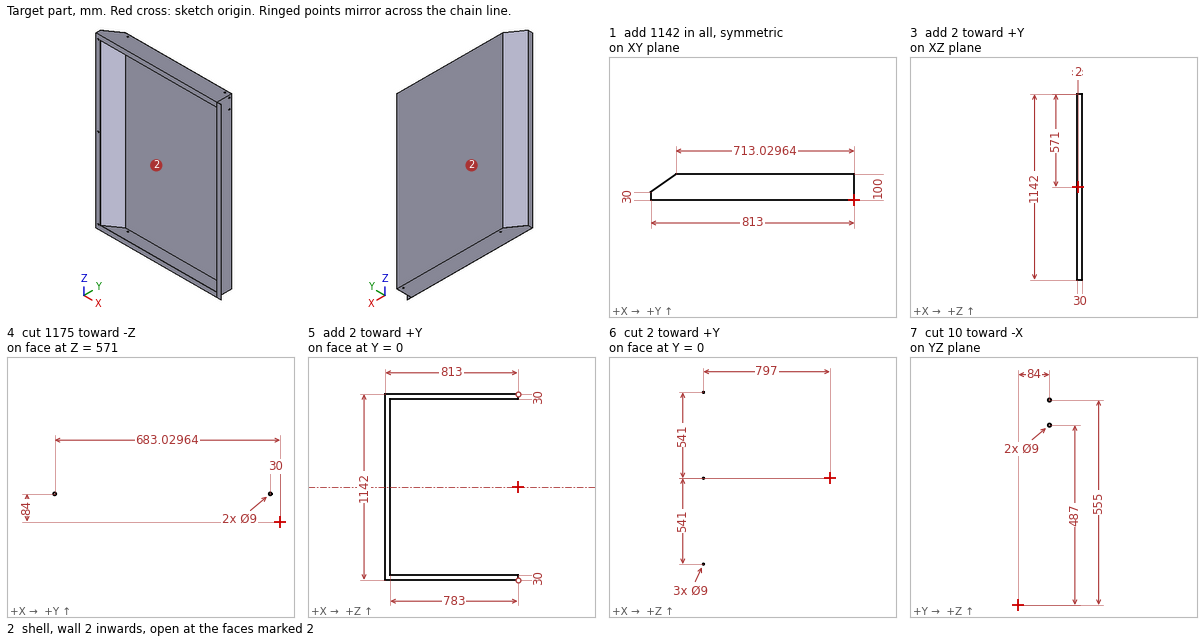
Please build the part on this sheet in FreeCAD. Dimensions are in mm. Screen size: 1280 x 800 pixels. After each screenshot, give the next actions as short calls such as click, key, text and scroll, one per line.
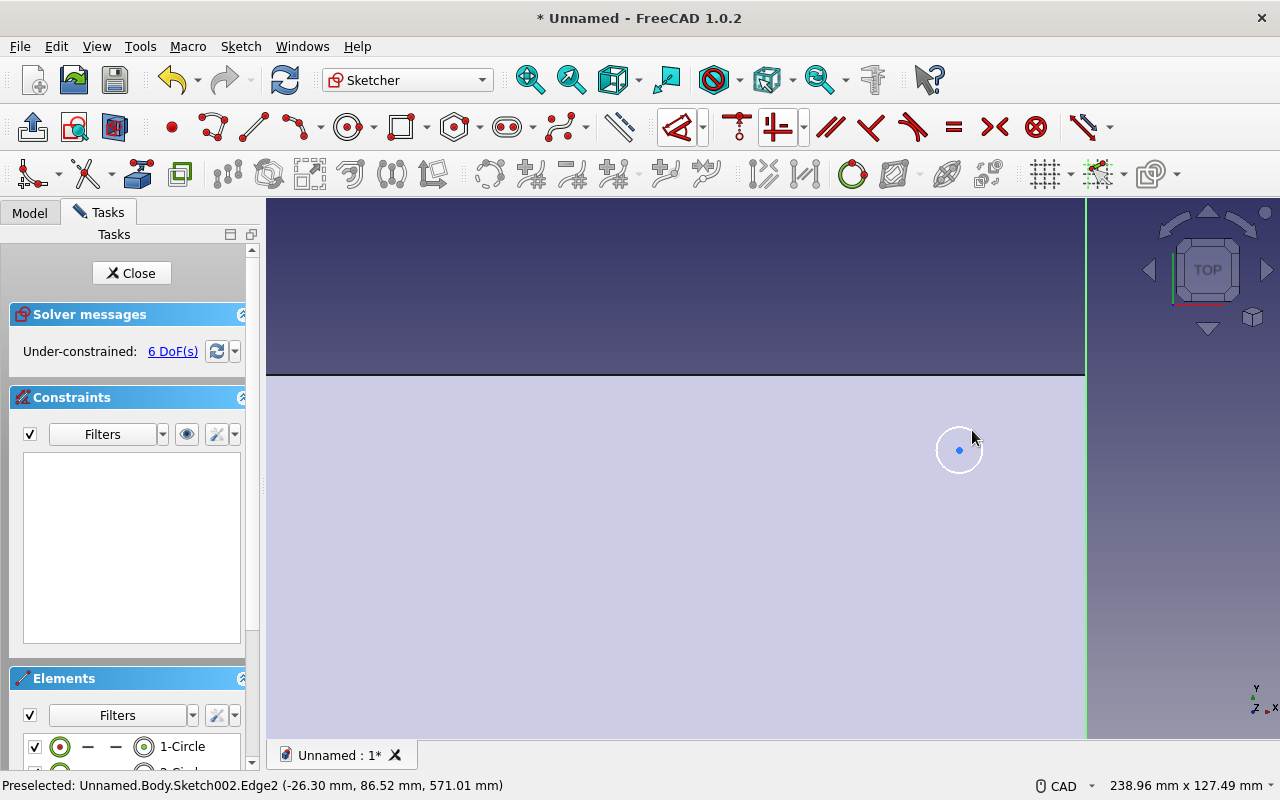
scroll(977, 432, down, 8)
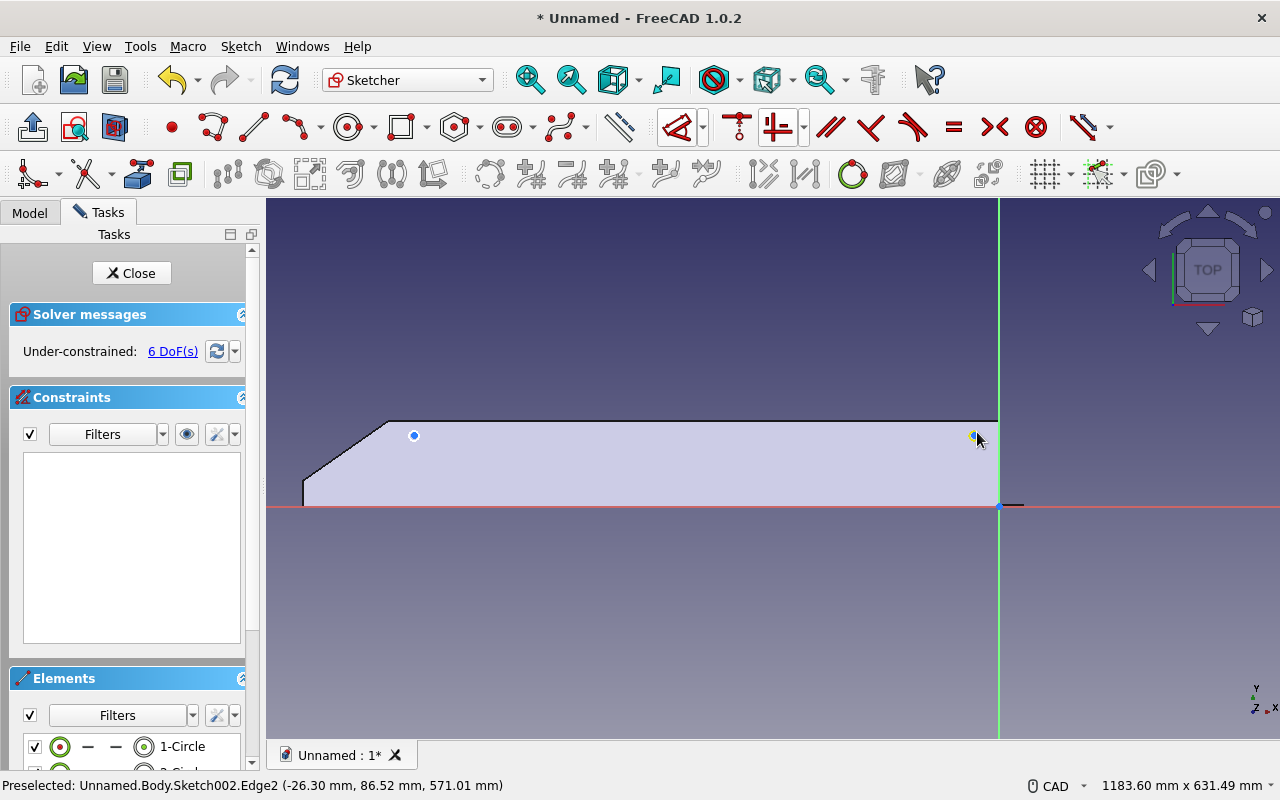
scroll(417, 432, up, 6)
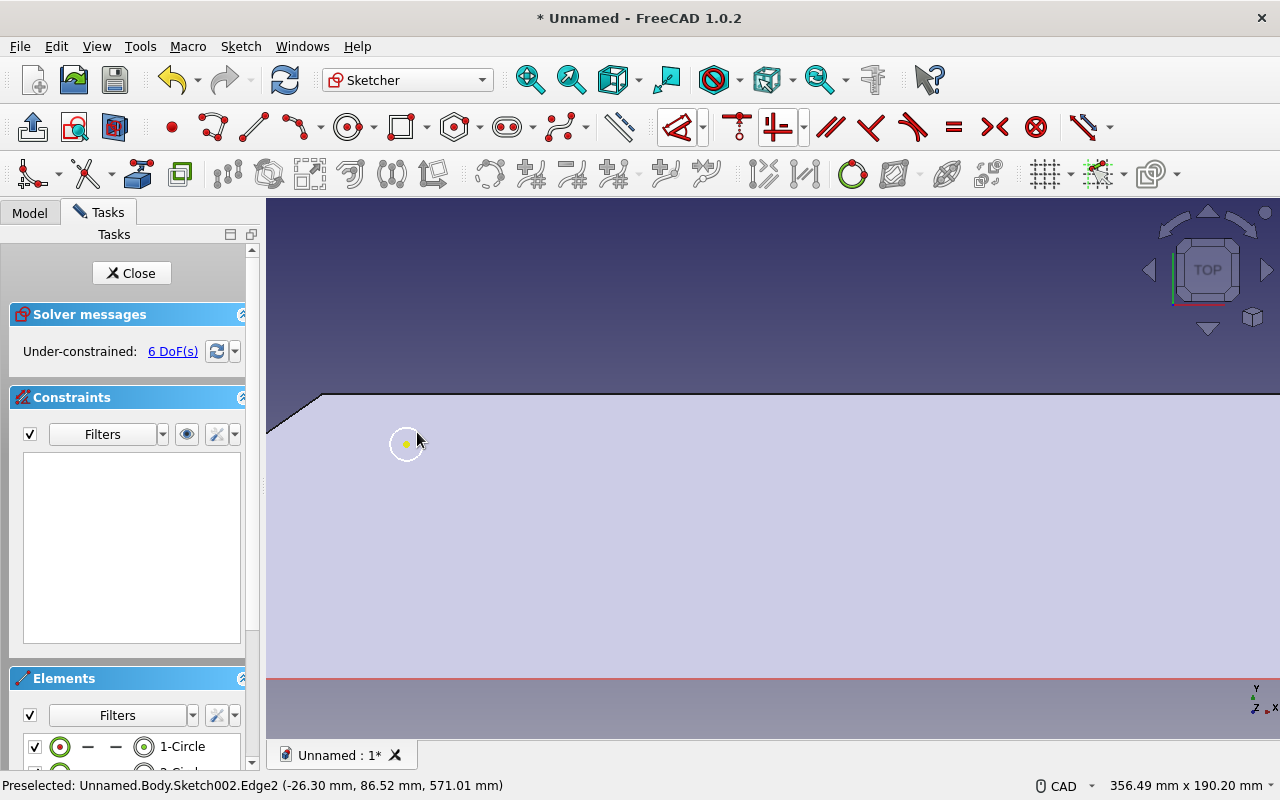
click(418, 433)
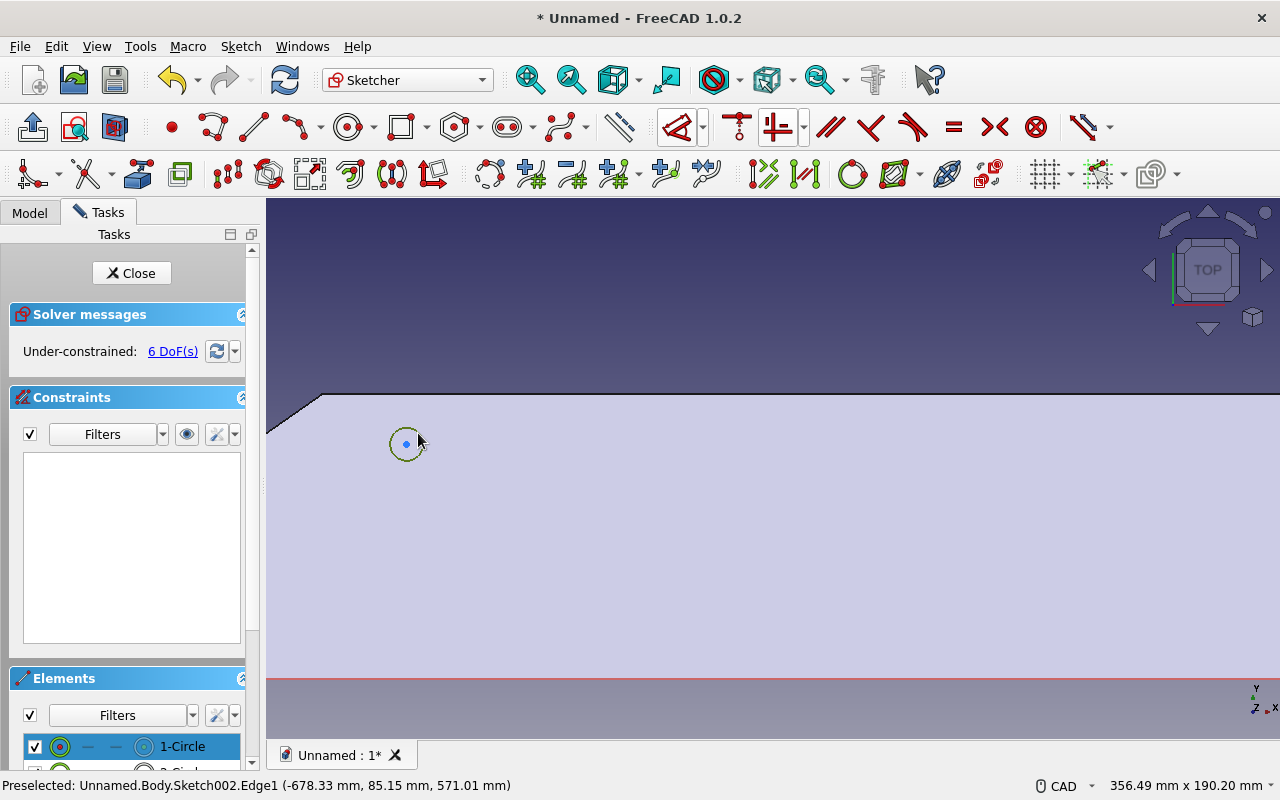
scroll(416, 432, down, 6)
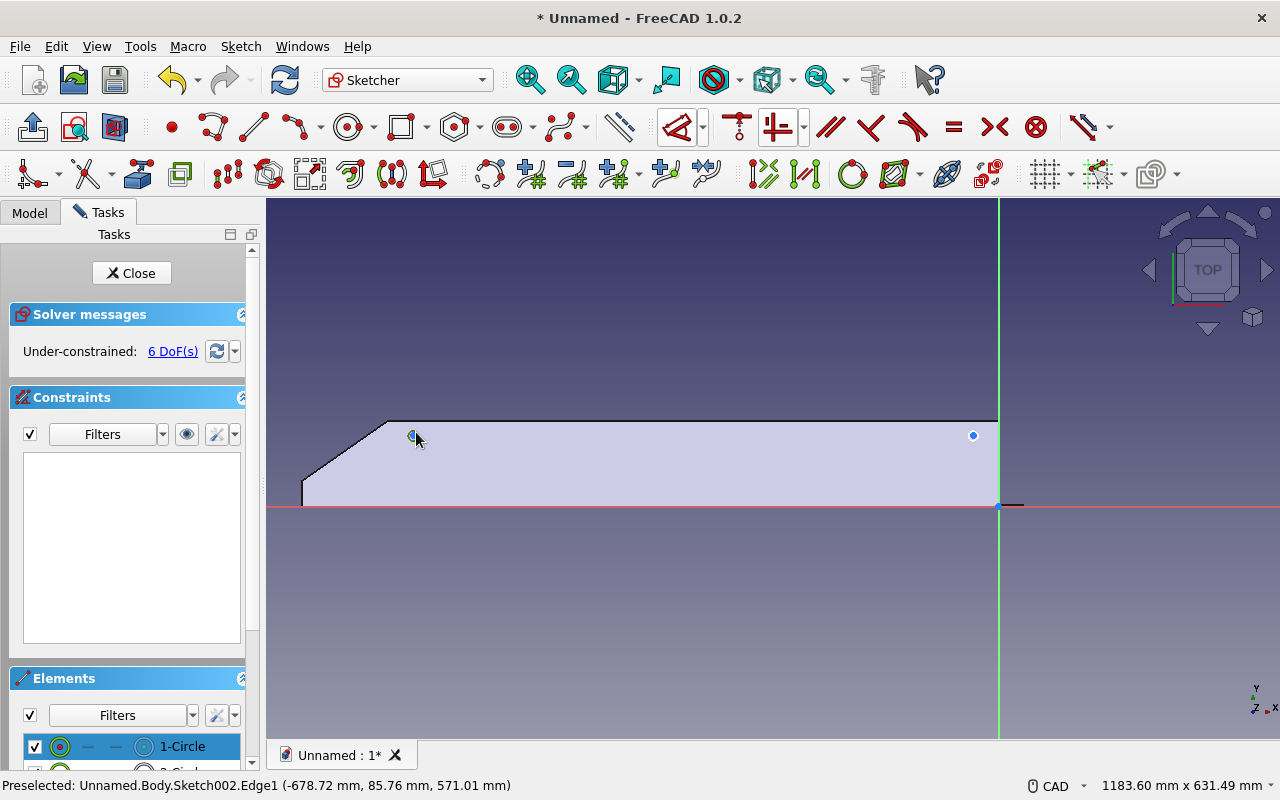
scroll(977, 433, up, 6)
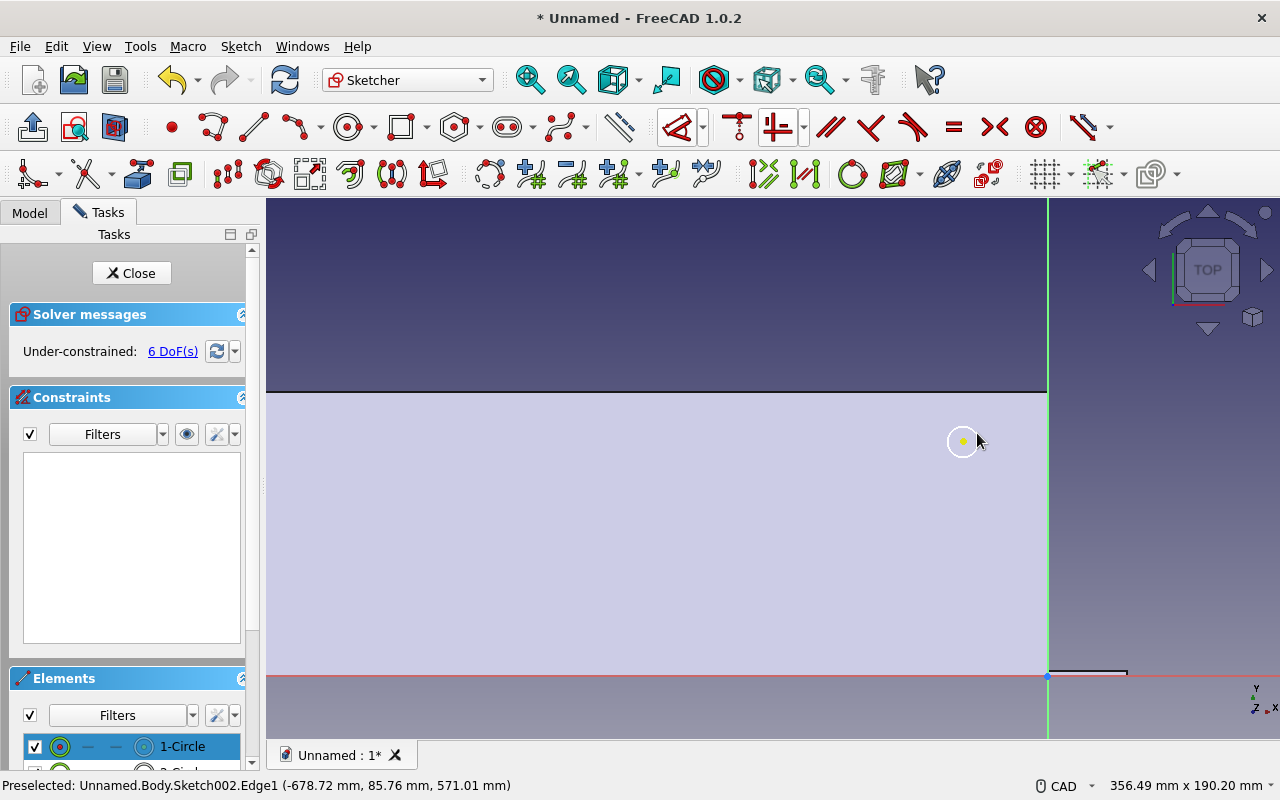
click(974, 431)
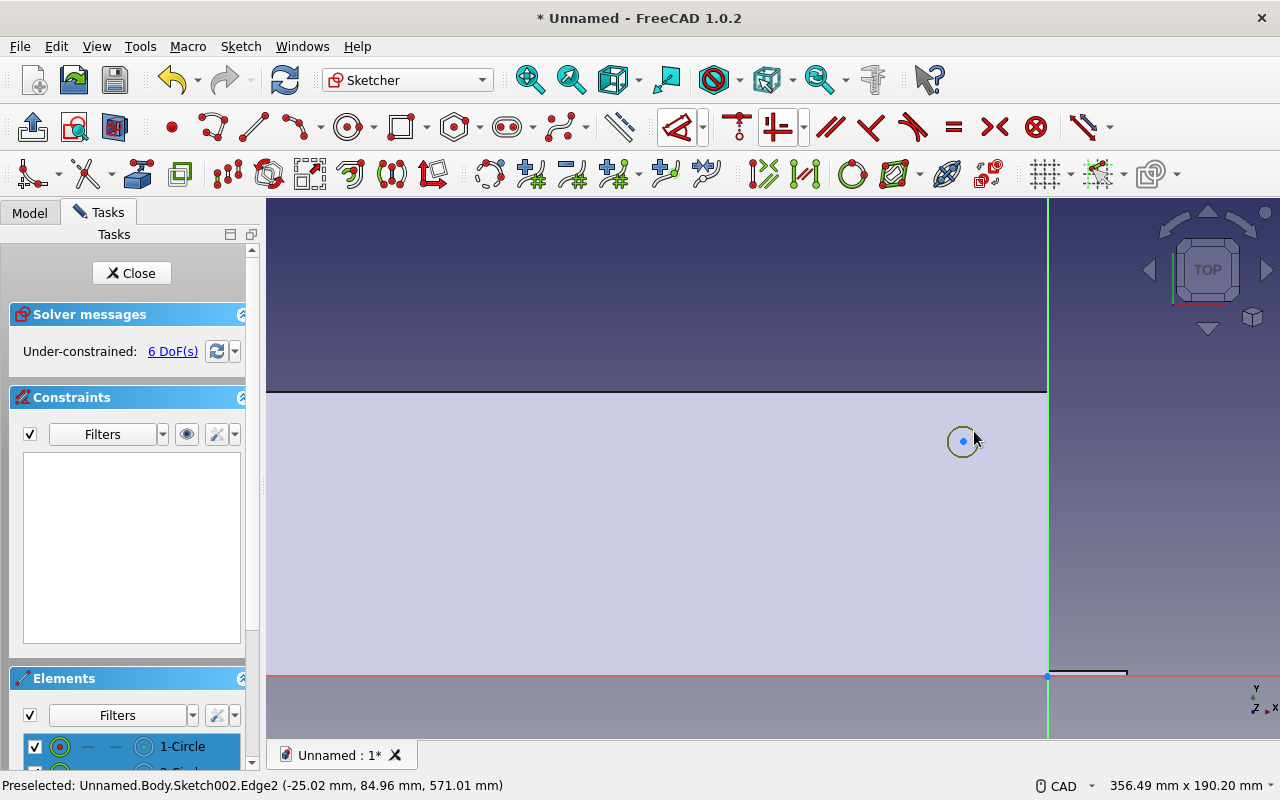
click(954, 128)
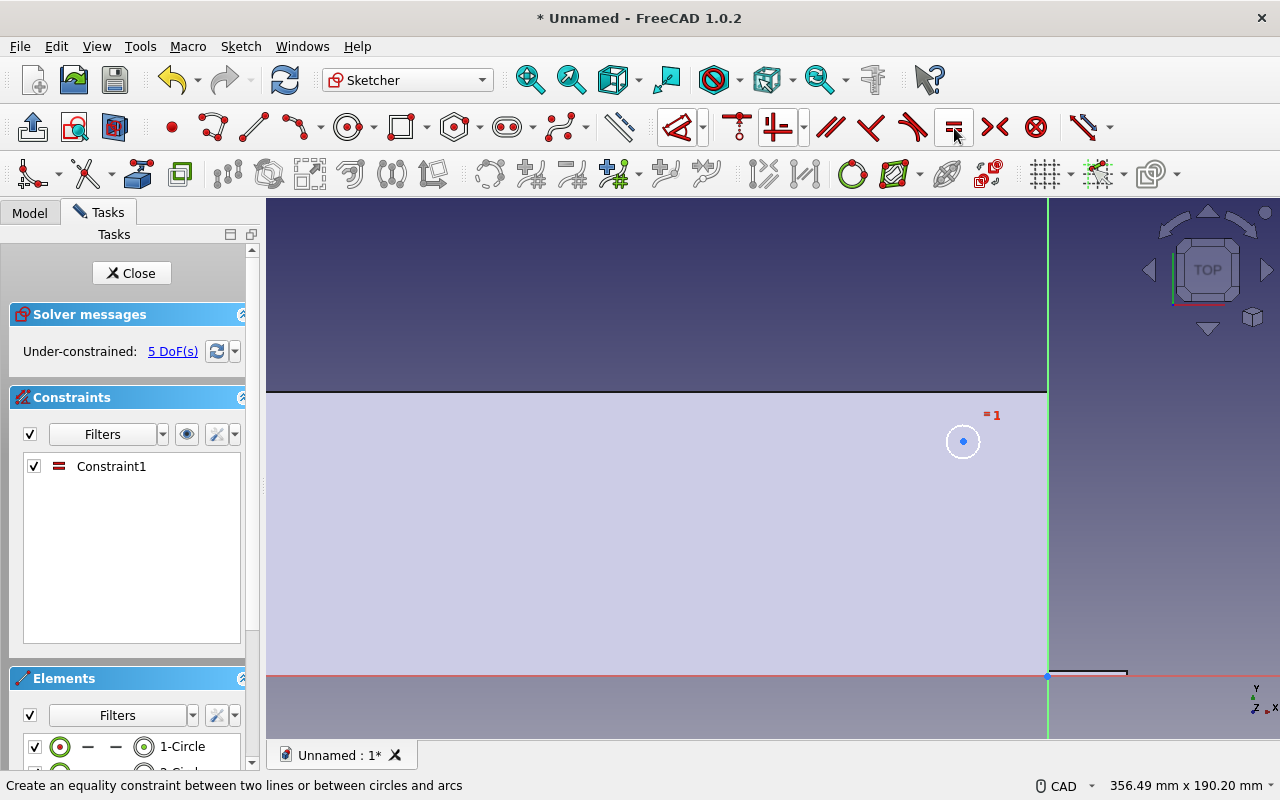
scroll(978, 433, down, 6)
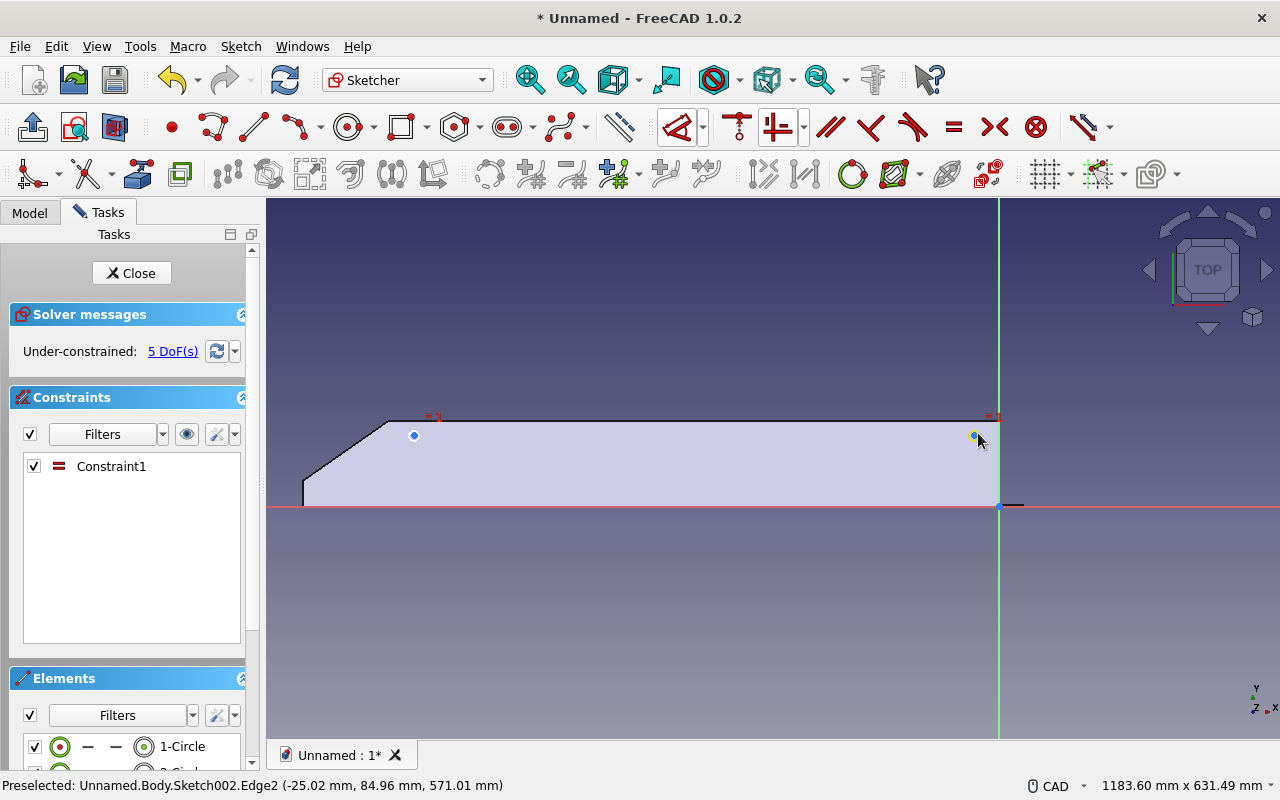
click(414, 436)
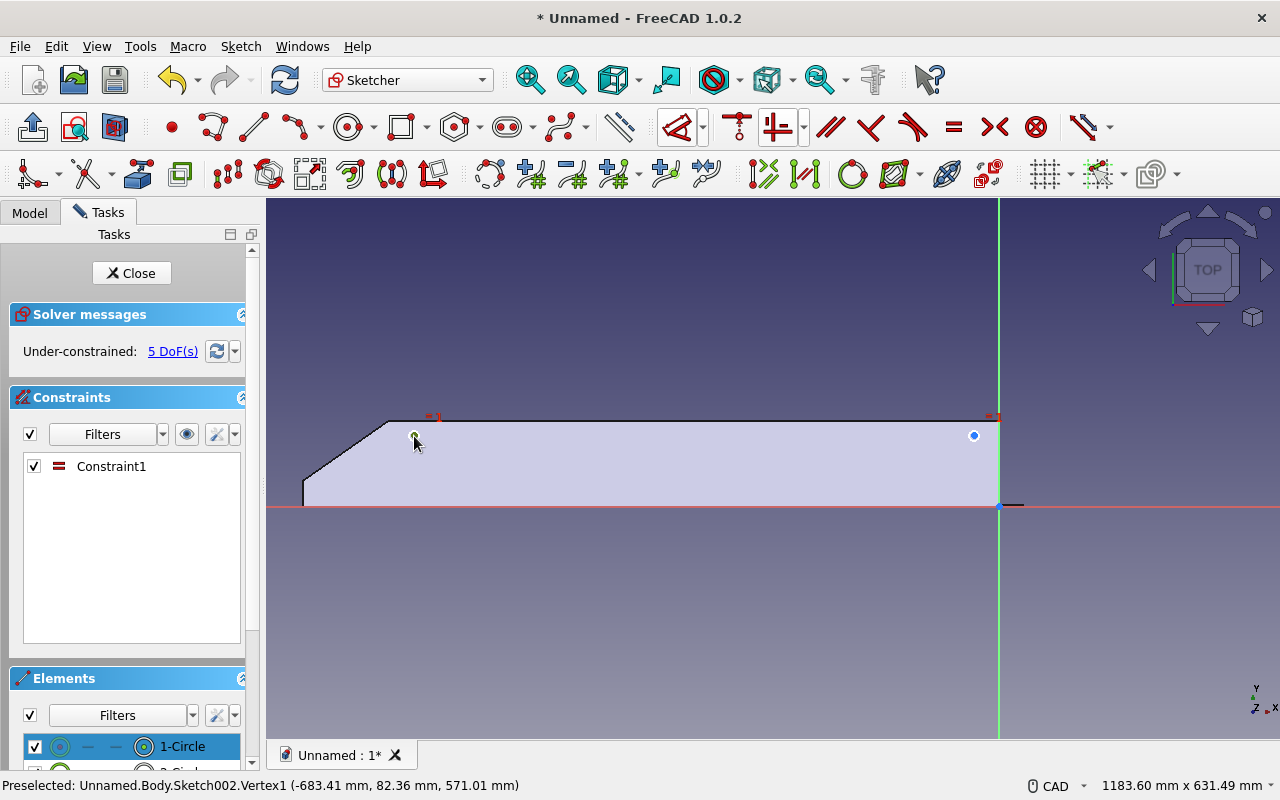
click(974, 436)